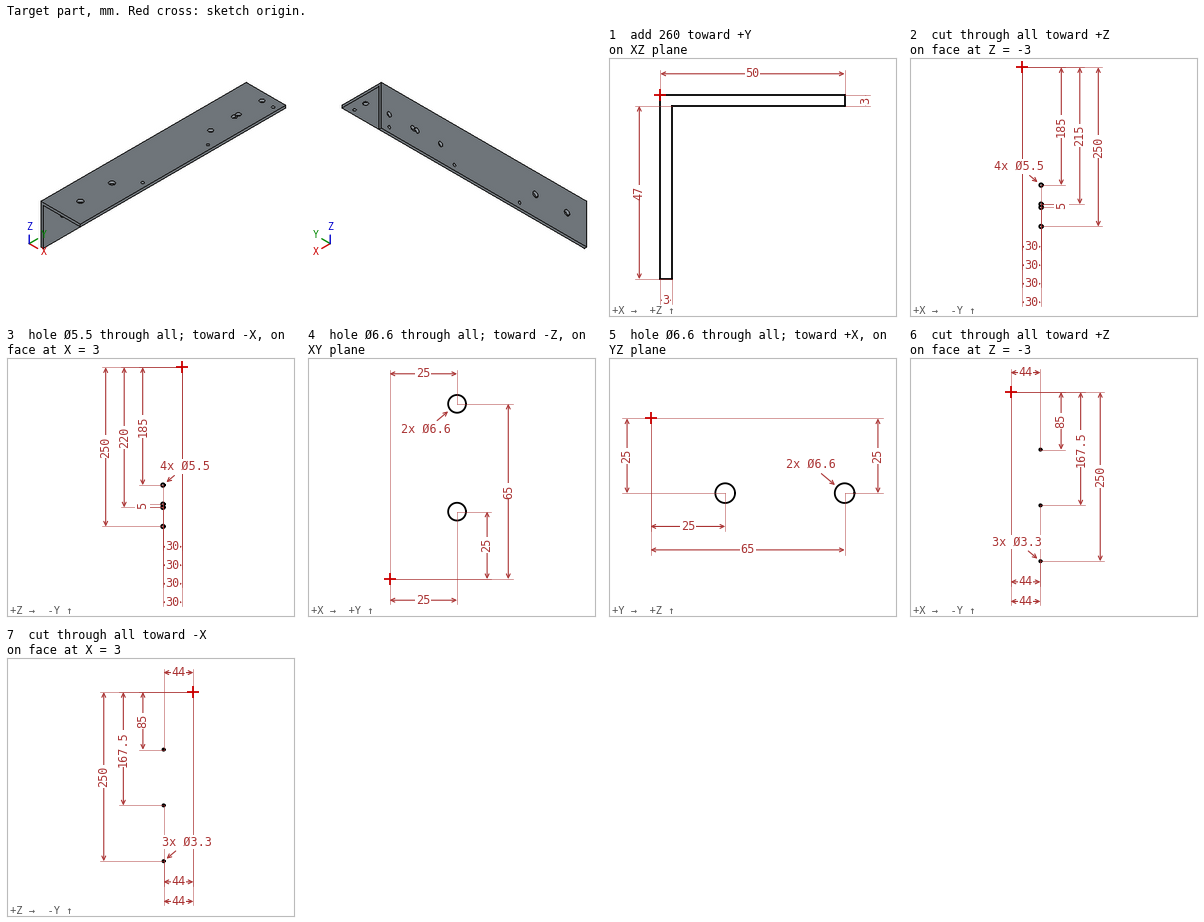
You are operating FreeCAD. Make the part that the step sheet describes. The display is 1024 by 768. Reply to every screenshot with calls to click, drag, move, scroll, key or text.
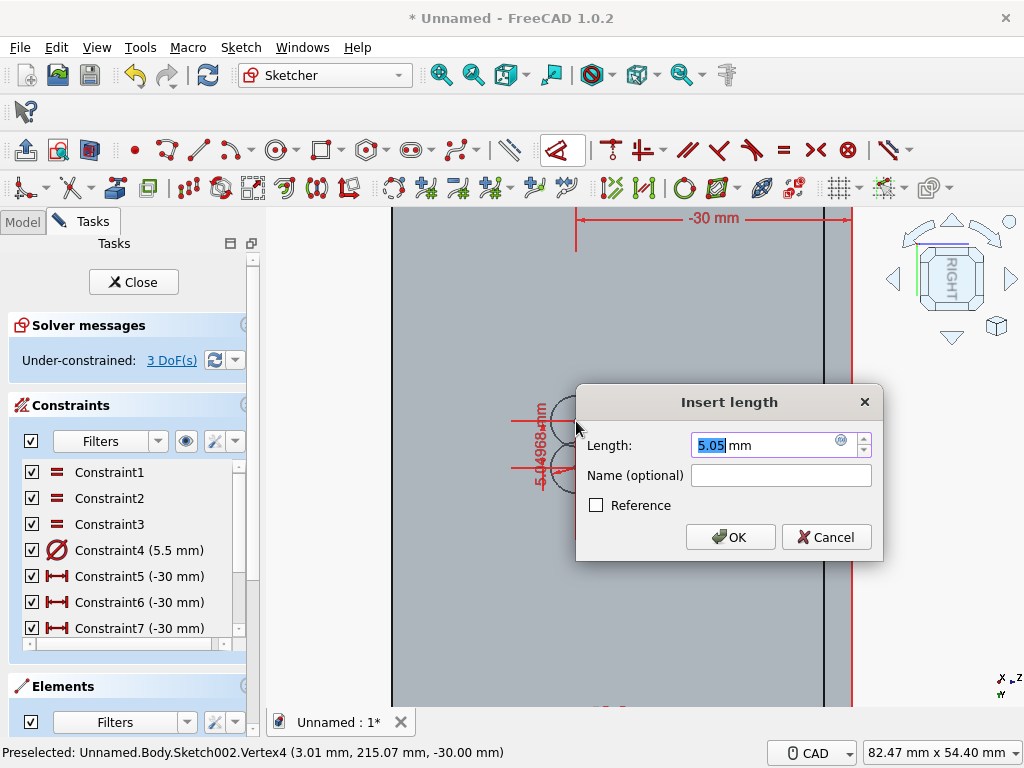
text(5)
key(Return)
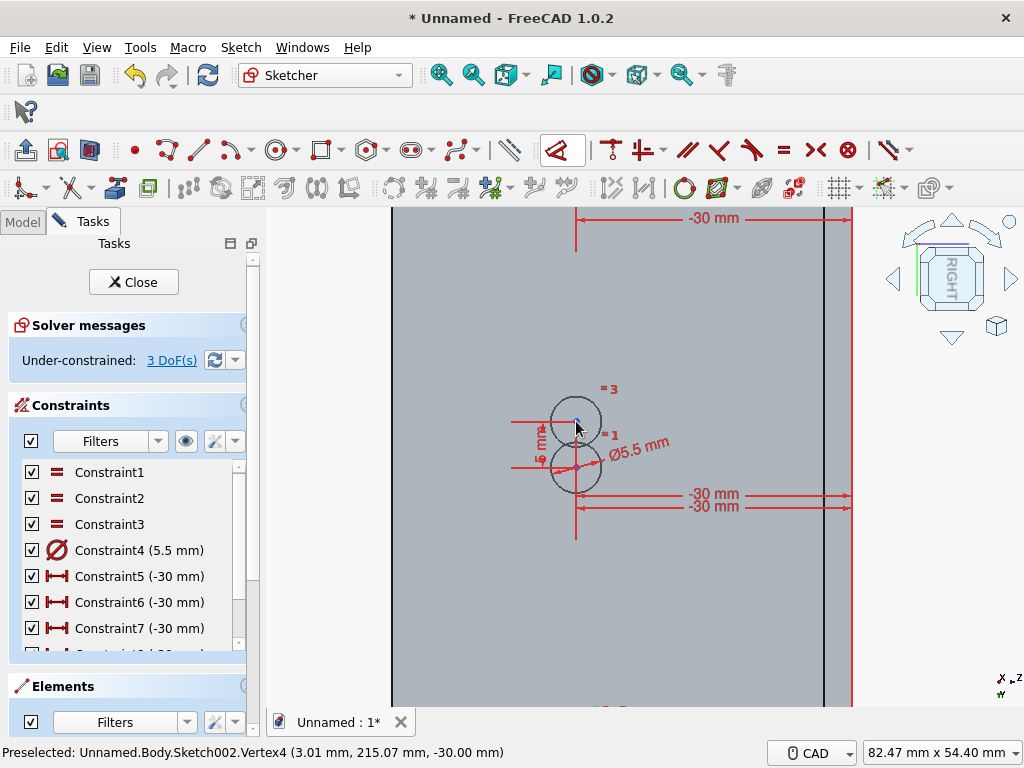
click(576, 468)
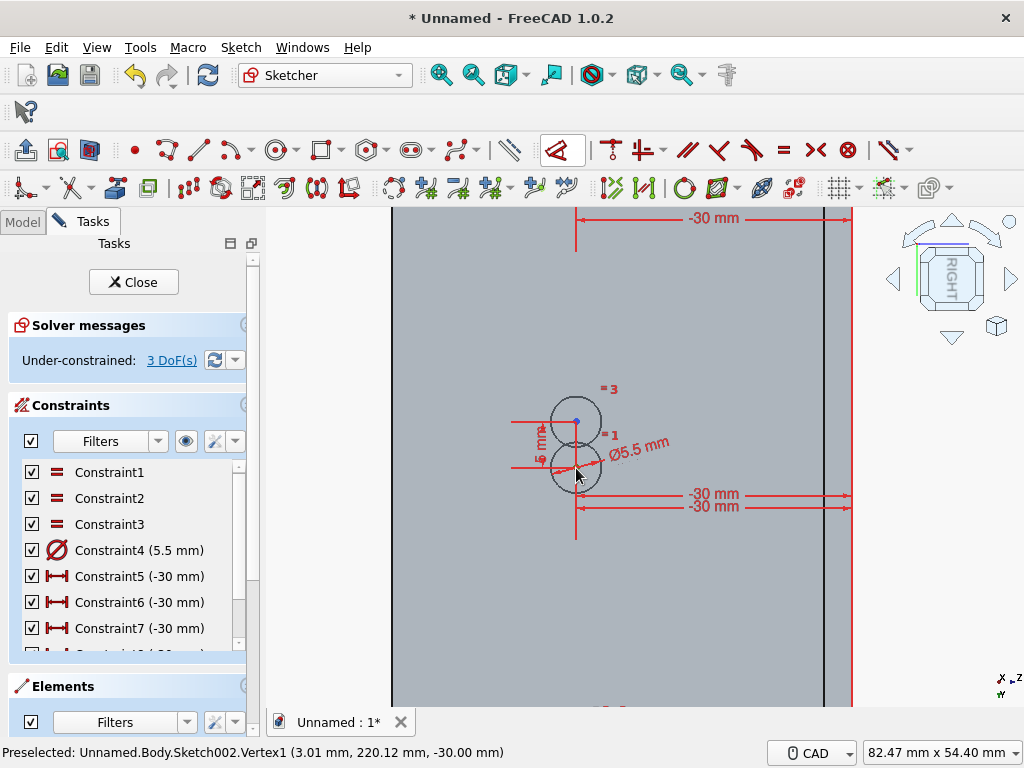
key(i)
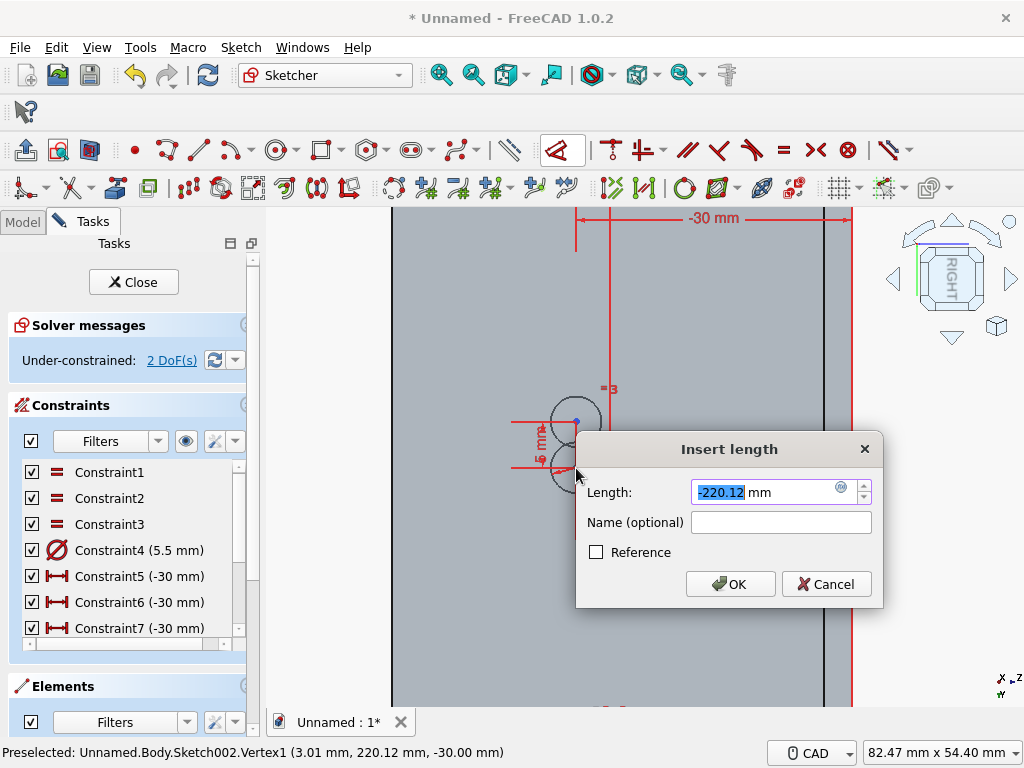
text(-220)
key(Return)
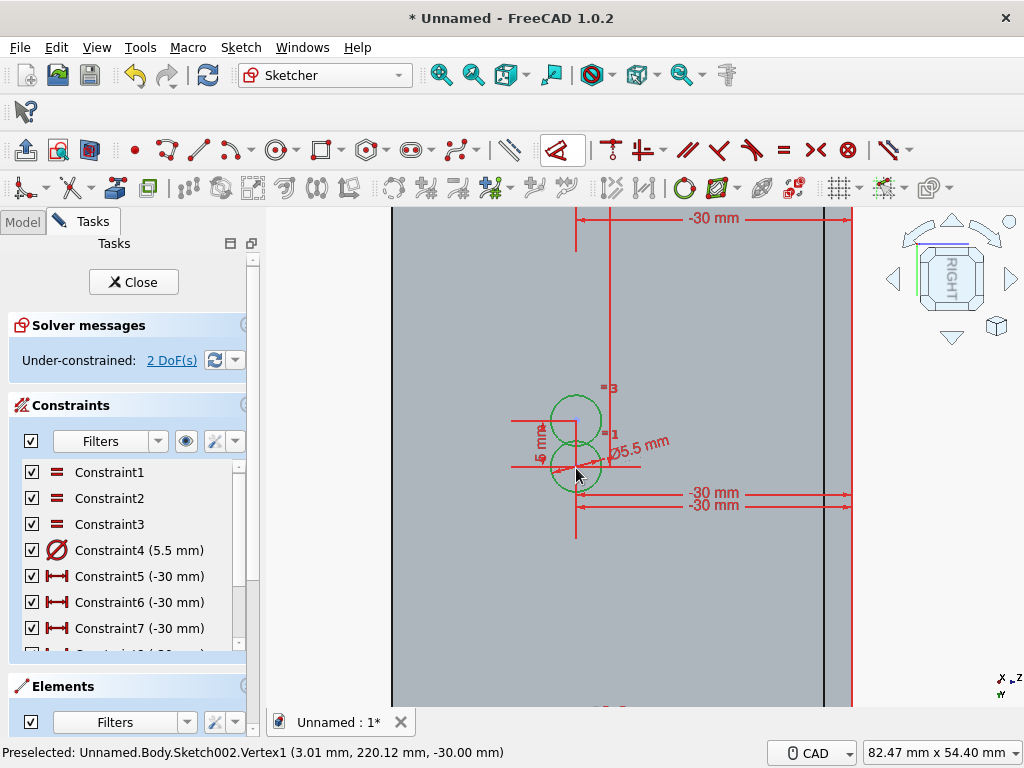
scroll(577, 468, down, 4)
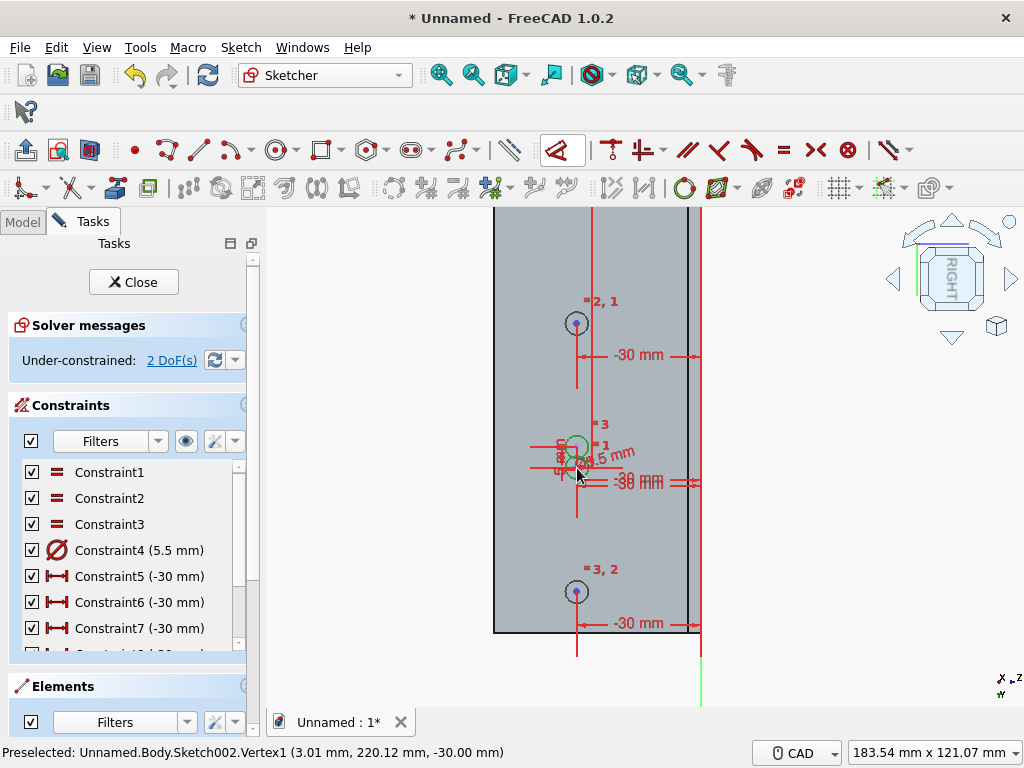
click(577, 324)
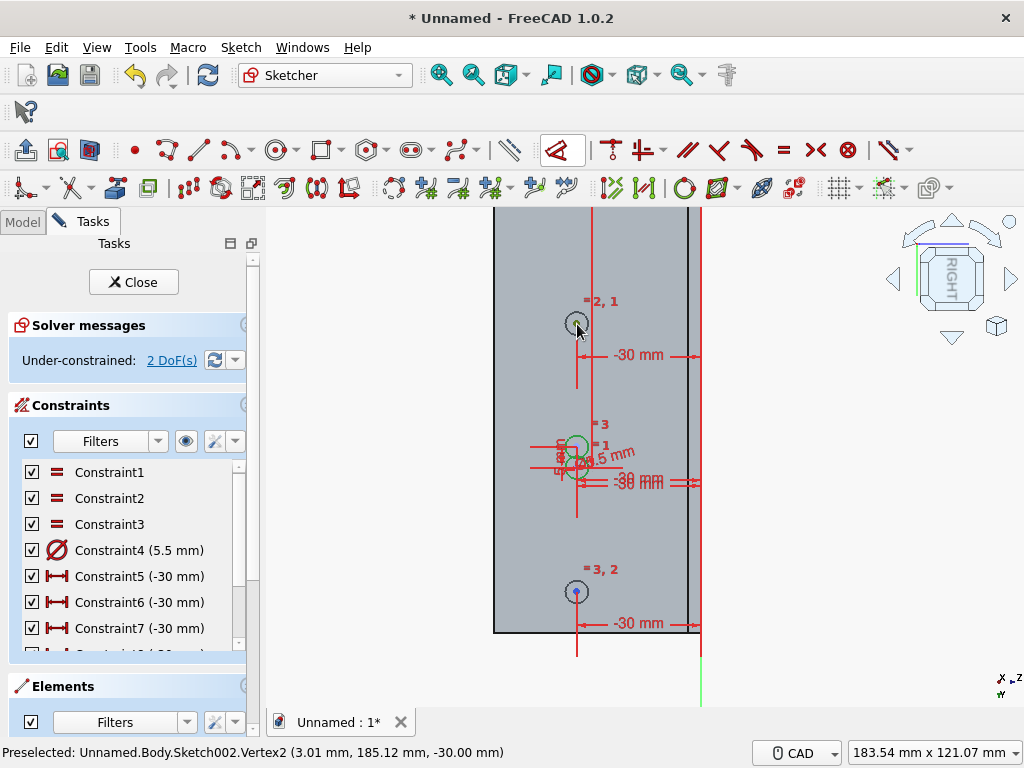
click(580, 150)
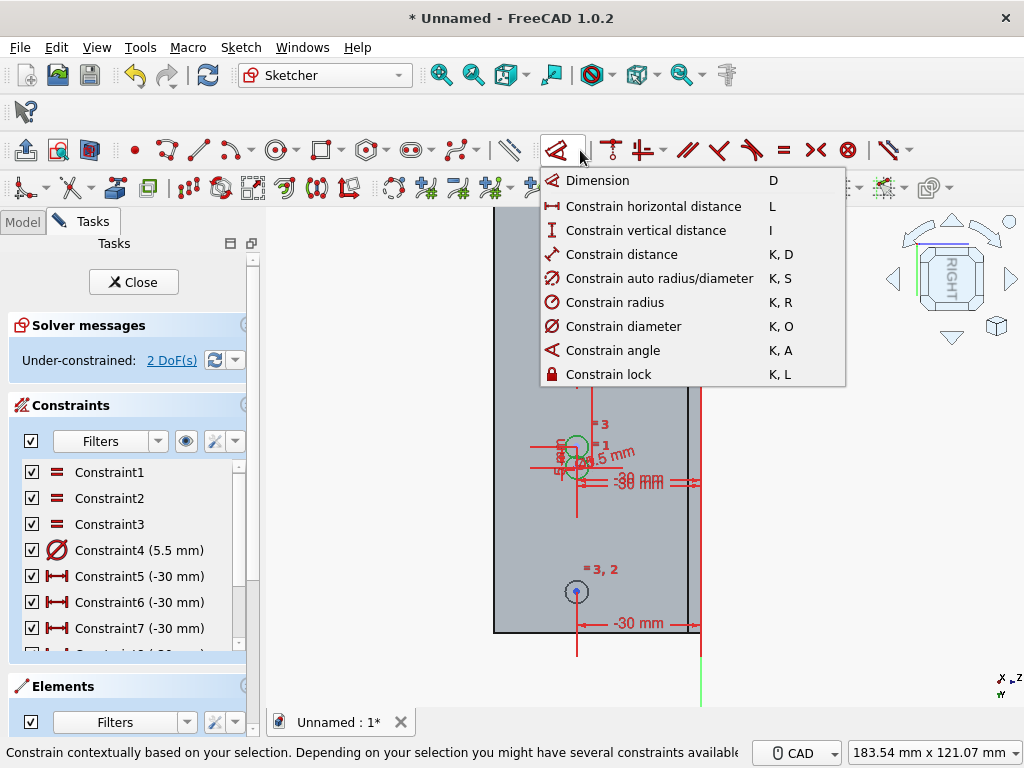
click(693, 230)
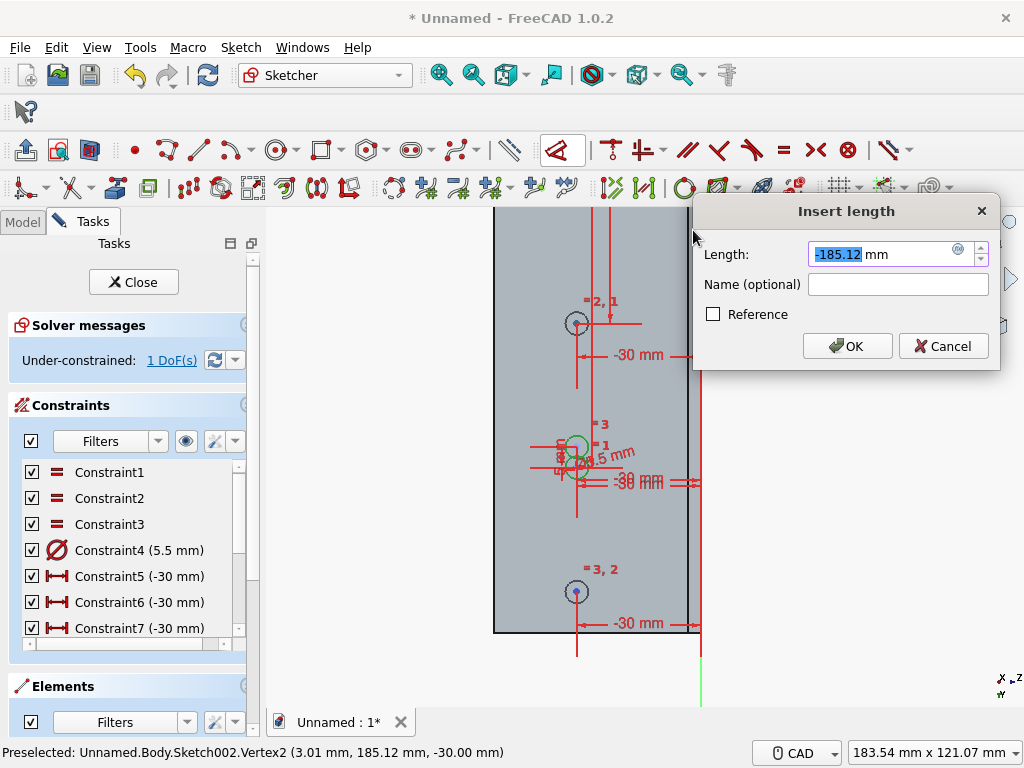
text(-185)
key(Return)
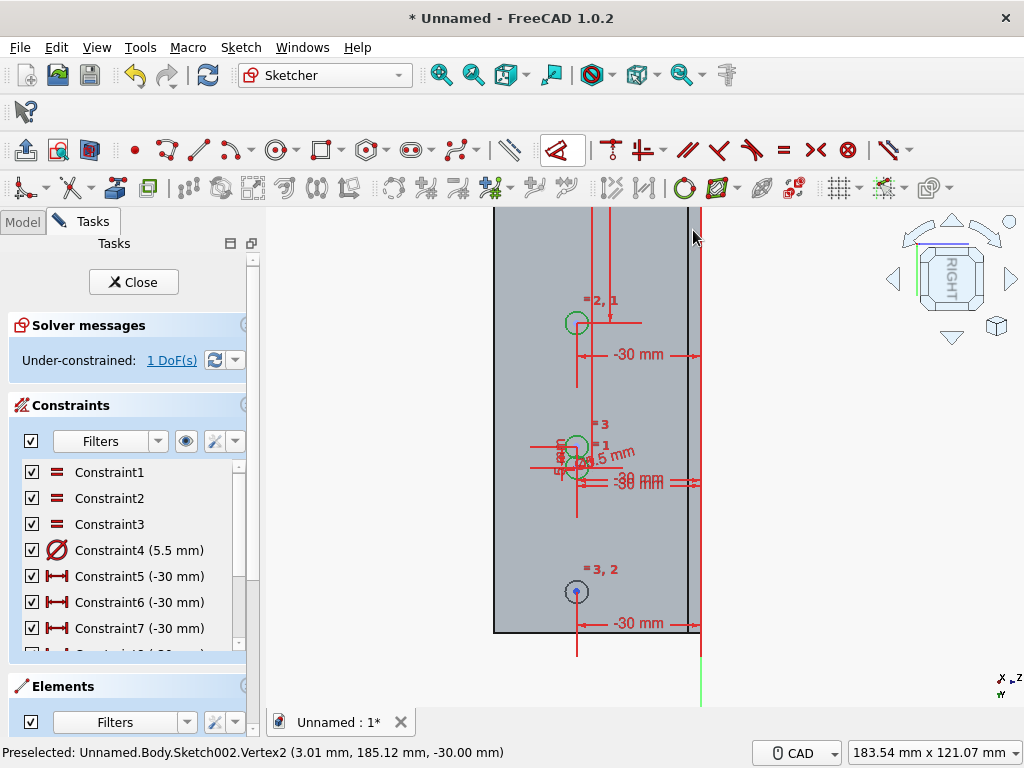
click(577, 592)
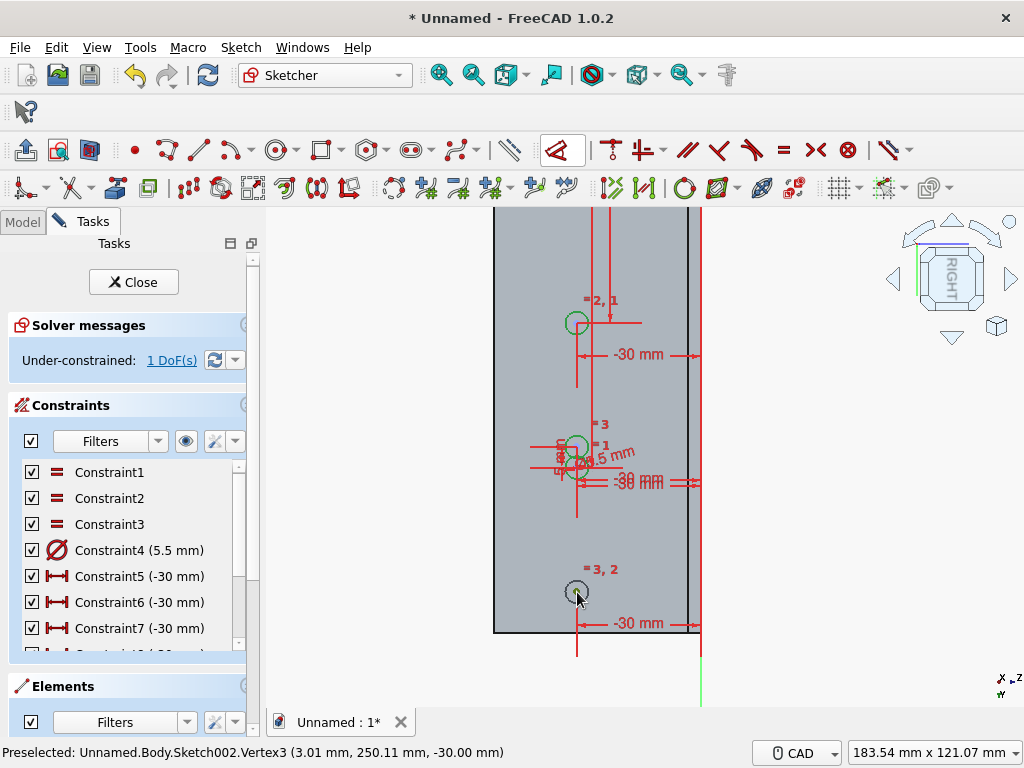
key(i)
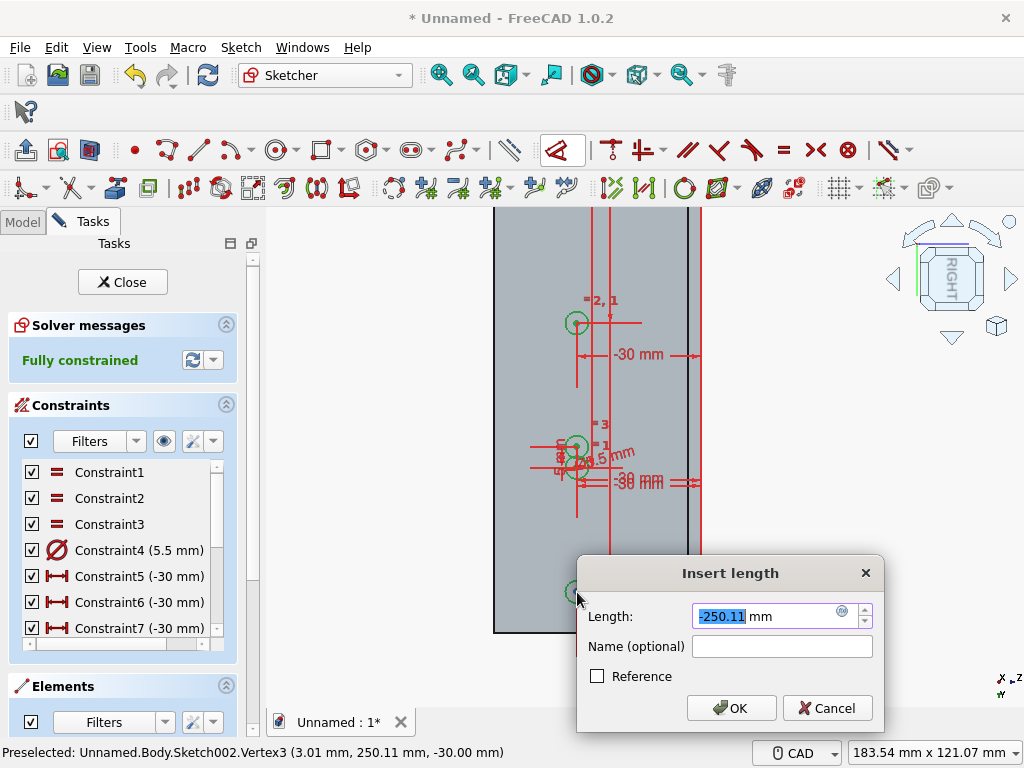
text(-250)
key(Return)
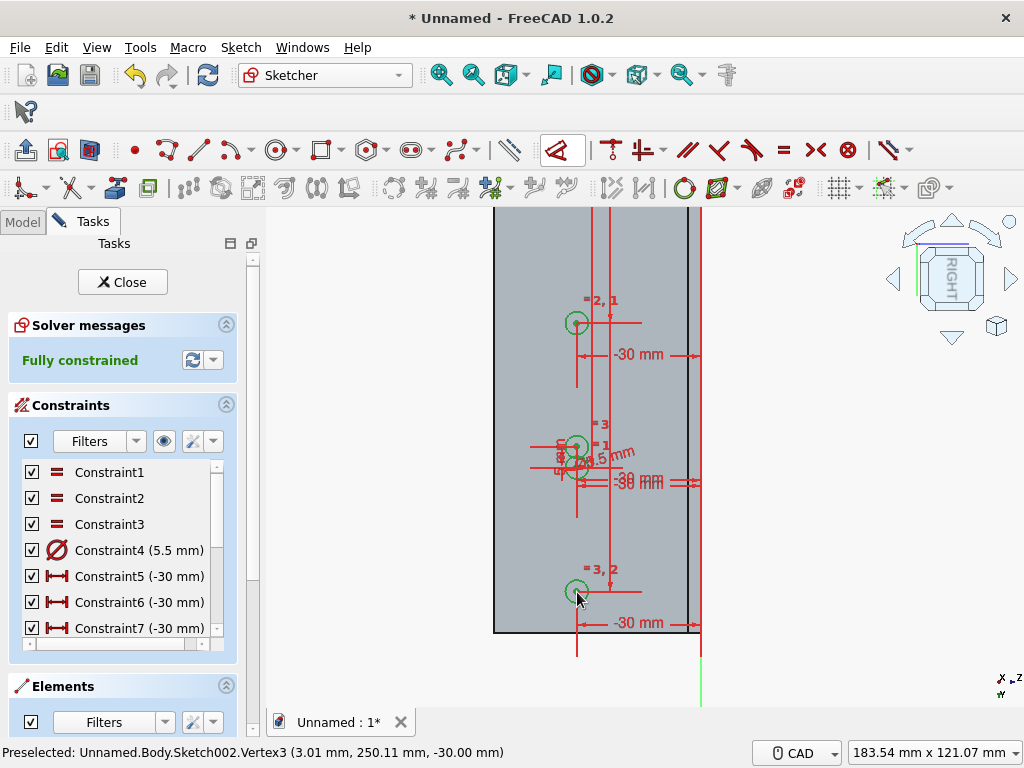
click(123, 282)